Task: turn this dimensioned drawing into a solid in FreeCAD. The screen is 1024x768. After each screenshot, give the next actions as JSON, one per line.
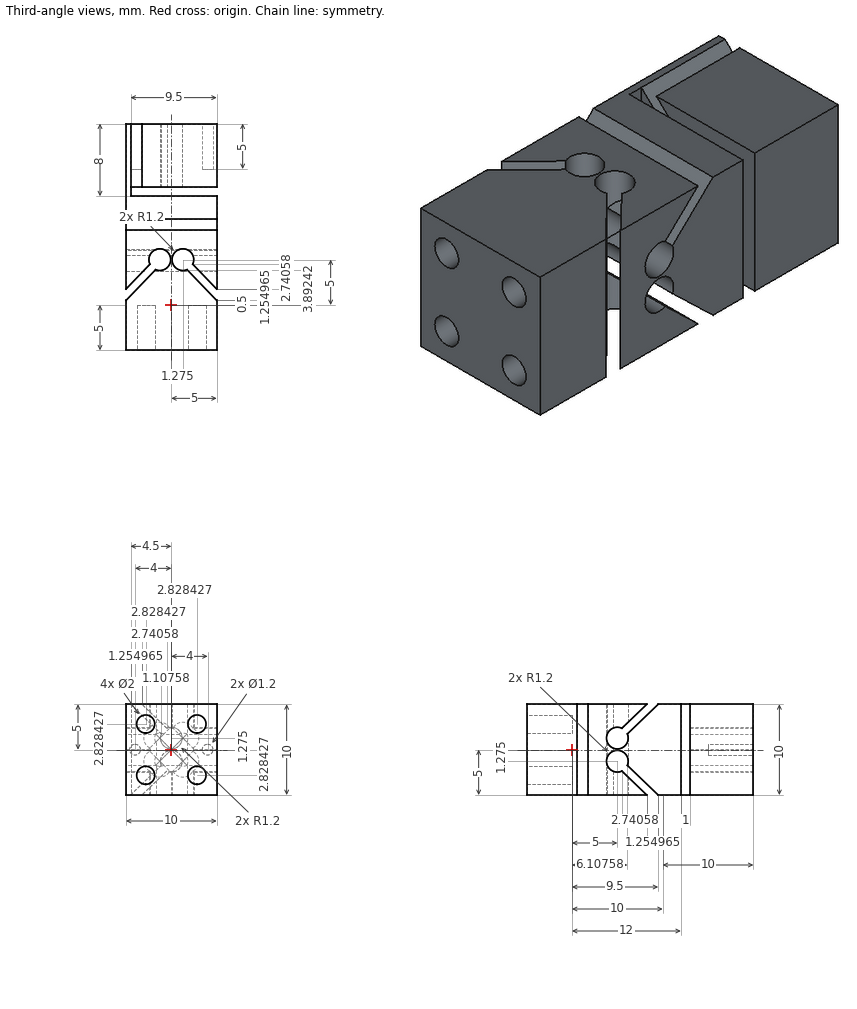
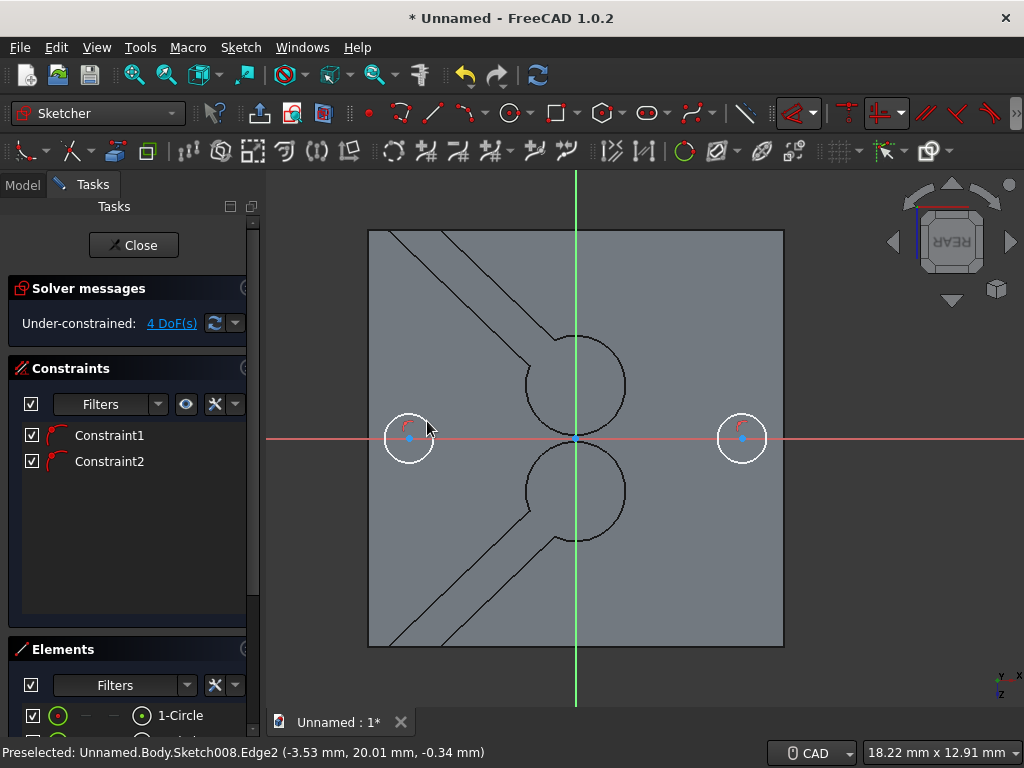
{"action": "left_click", "coordinate": [759, 421]}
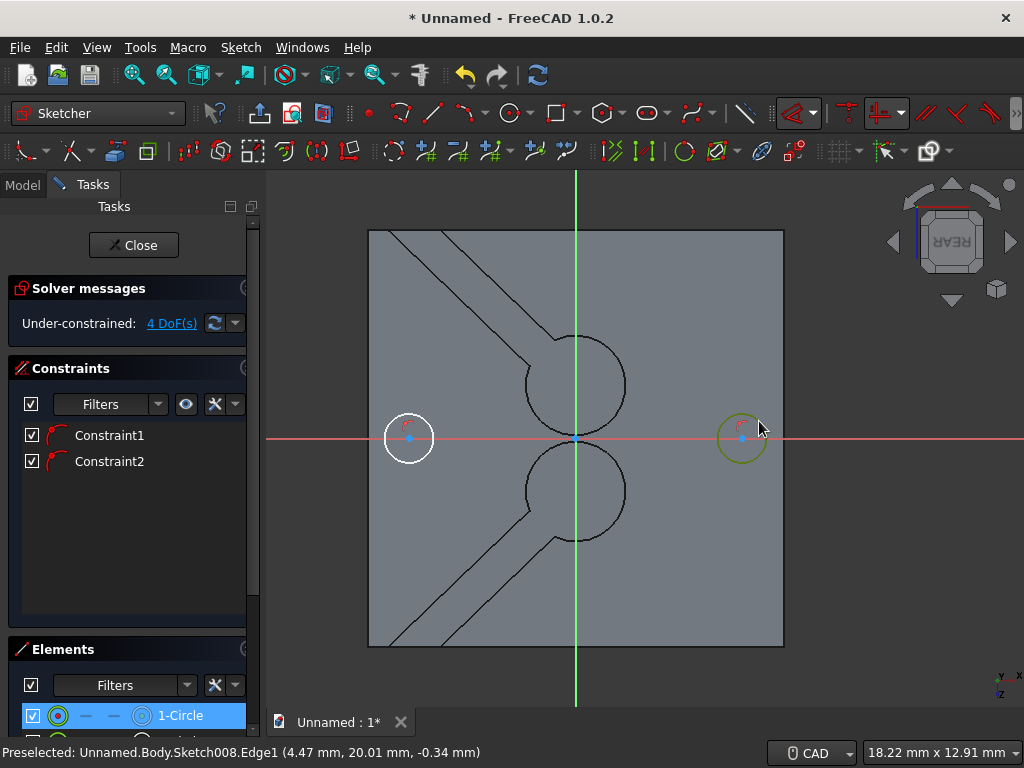
{"action": "left_click", "coordinate": [426, 421]}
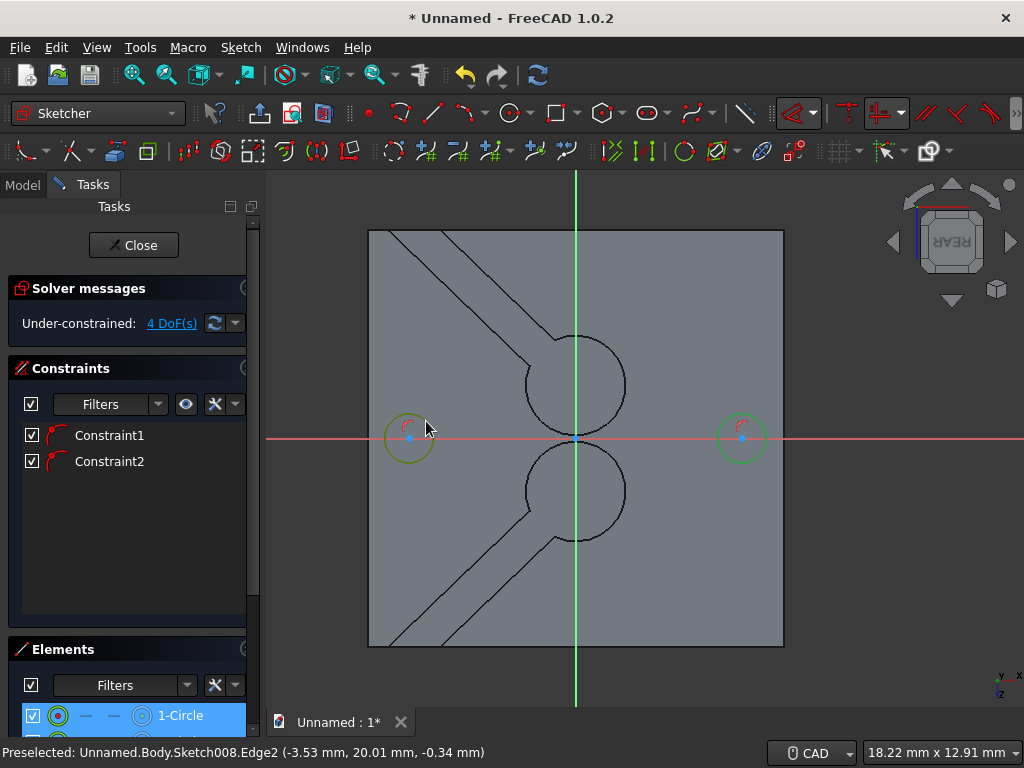
{"action": "key", "text": "e"}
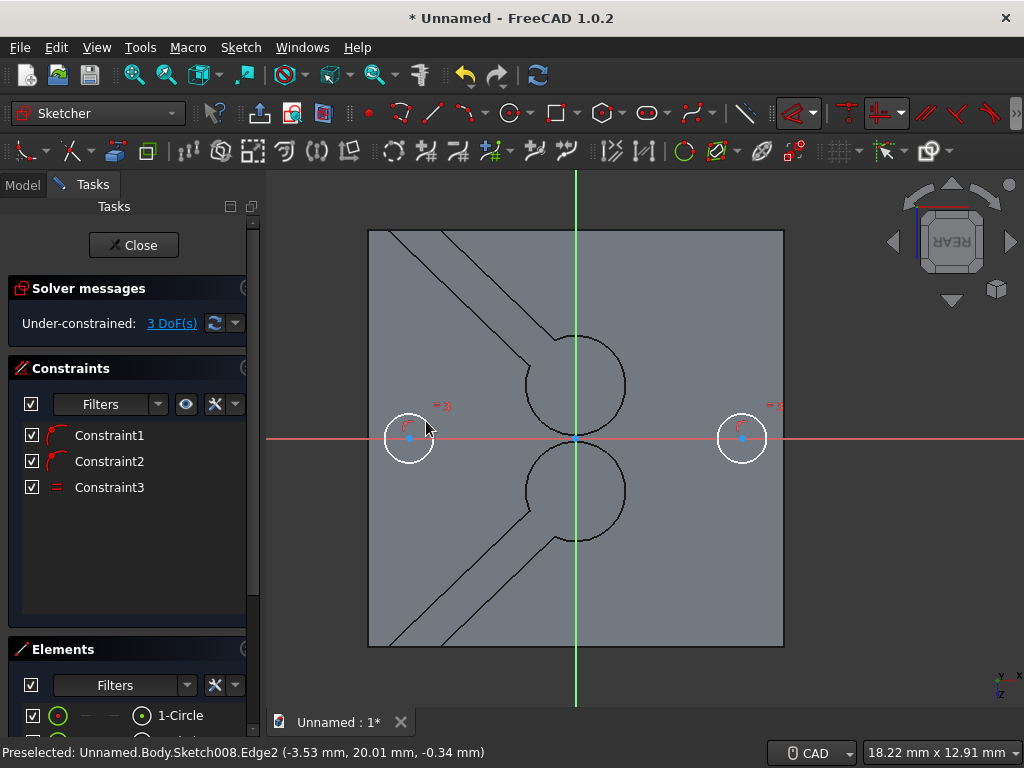
{"action": "left_click", "coordinate": [759, 421]}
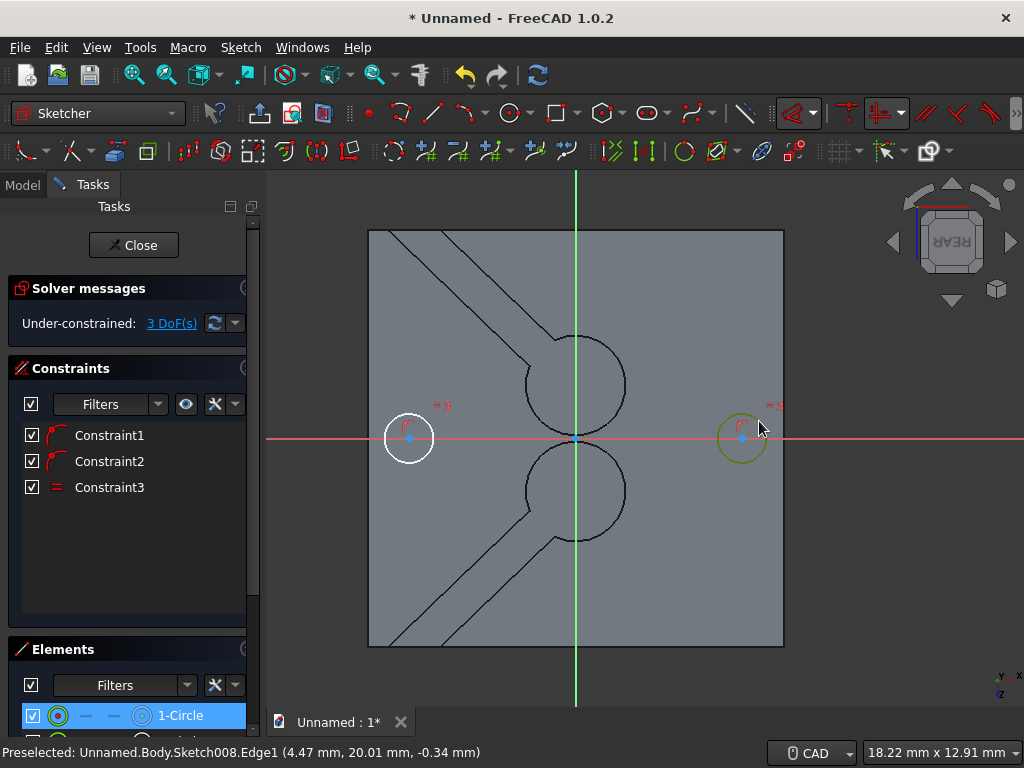
{"action": "left_click", "coordinate": [816, 114]}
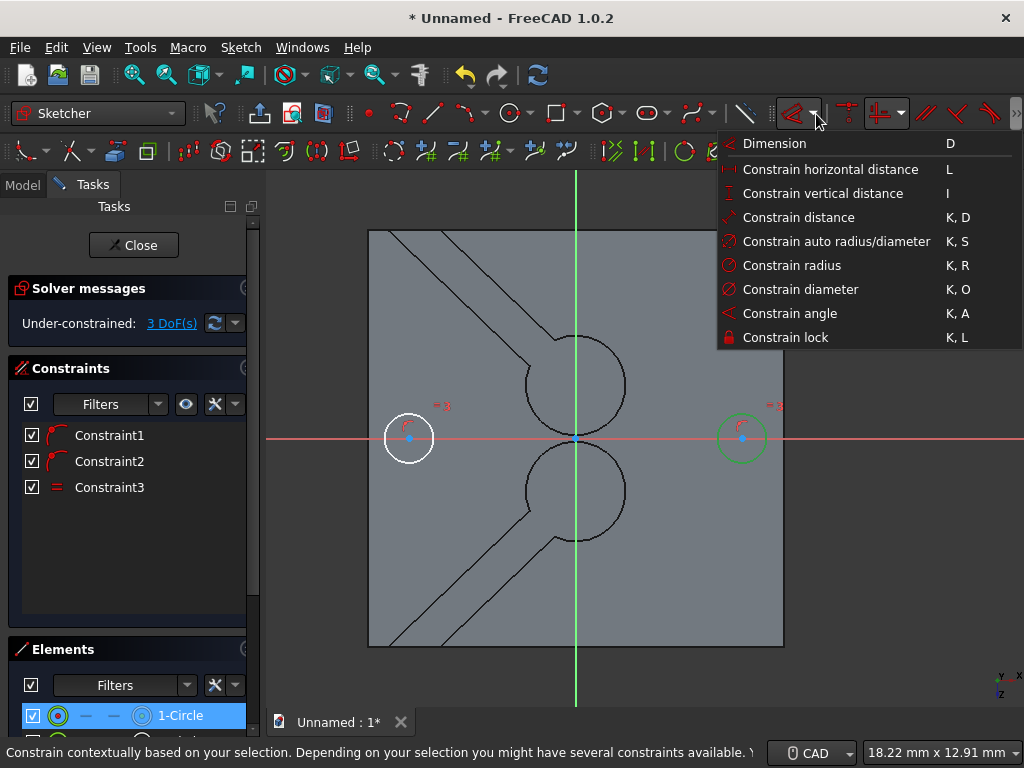
{"action": "left_click", "coordinate": [870, 289]}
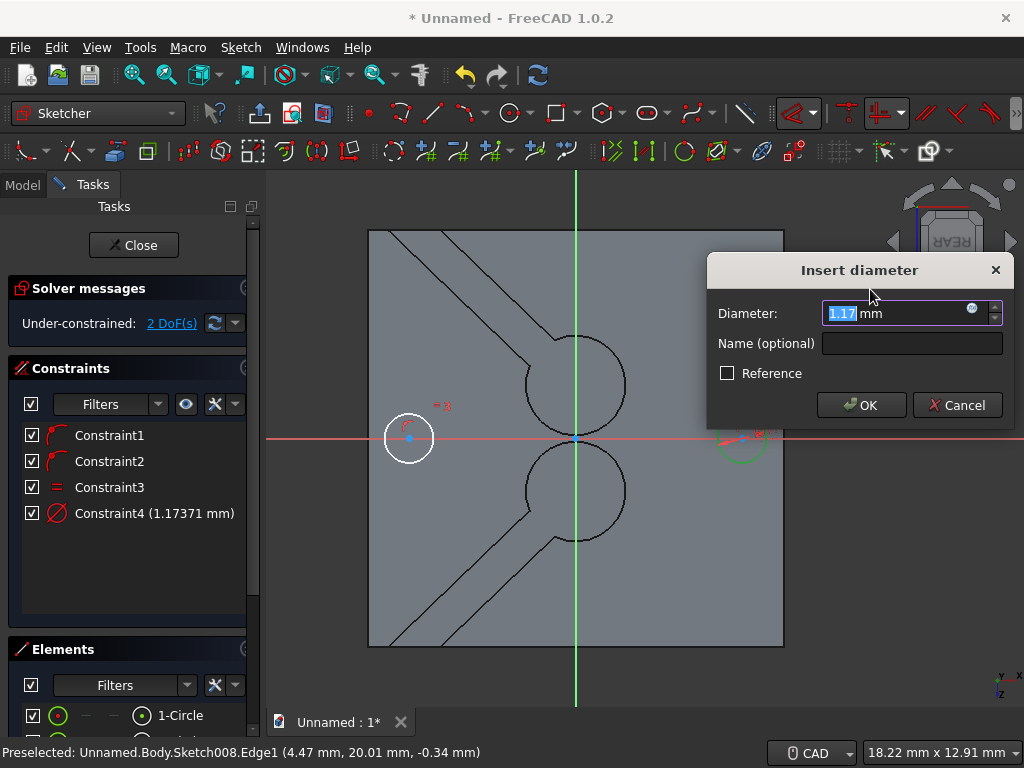
{"action": "type", "text": "1.2"}
{"action": "key", "text": "Return"}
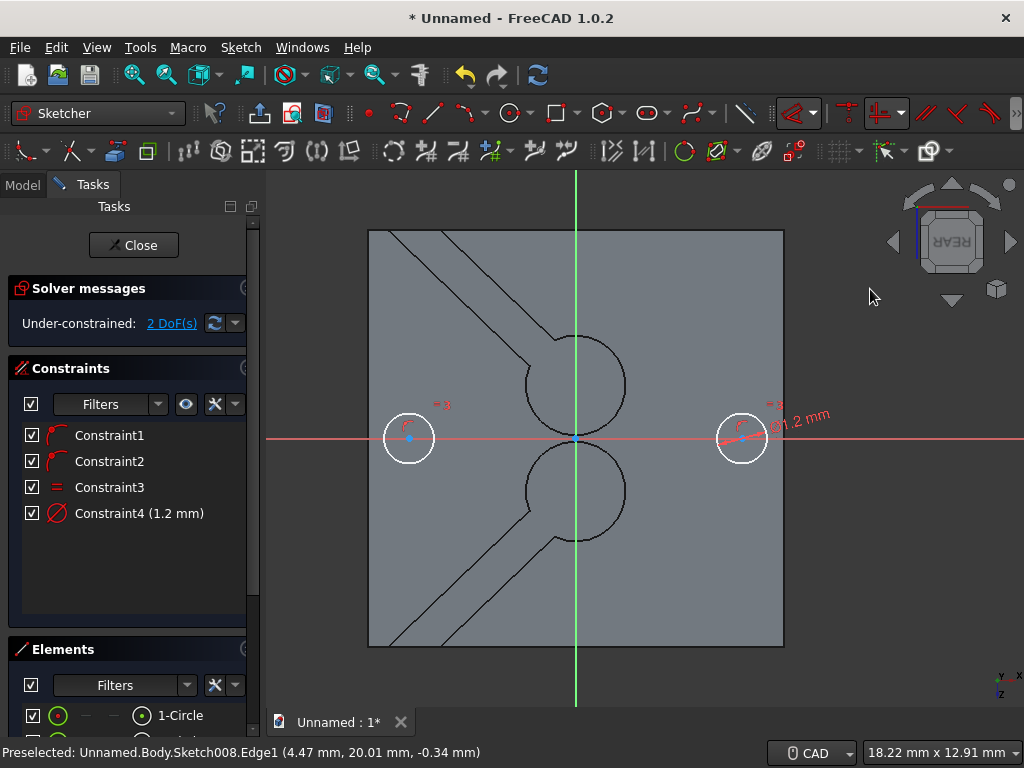
{"action": "left_click", "coordinate": [742, 438]}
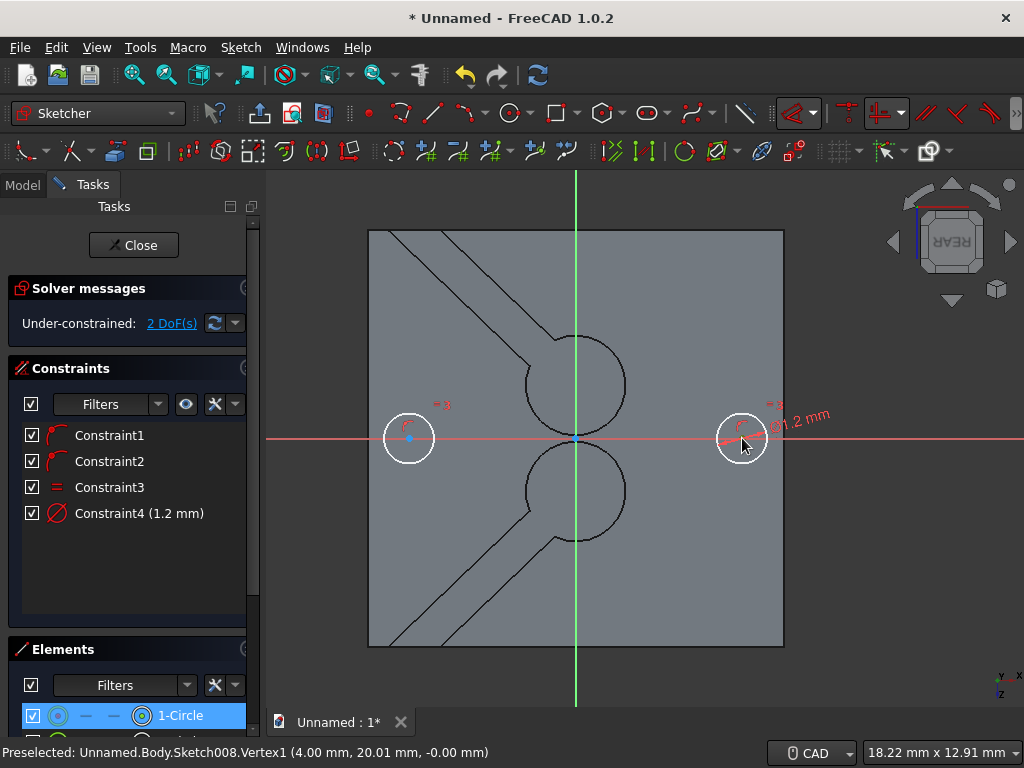
{"action": "key", "text": "l"}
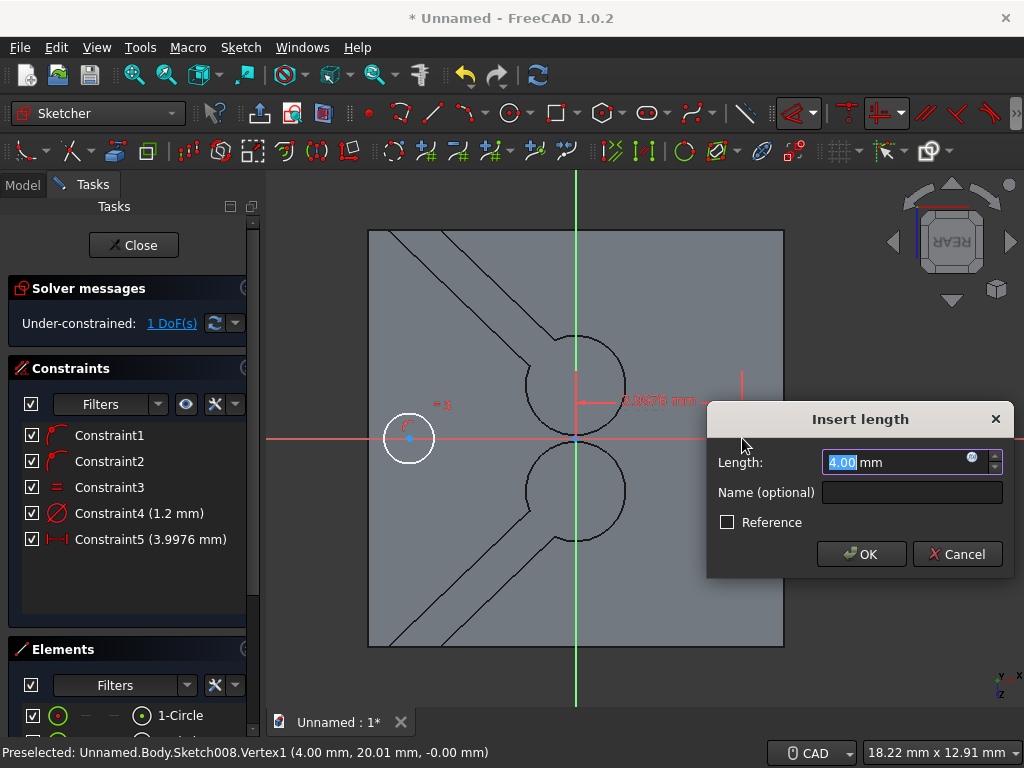
{"action": "type", "text": "4"}
{"action": "key", "text": "Return"}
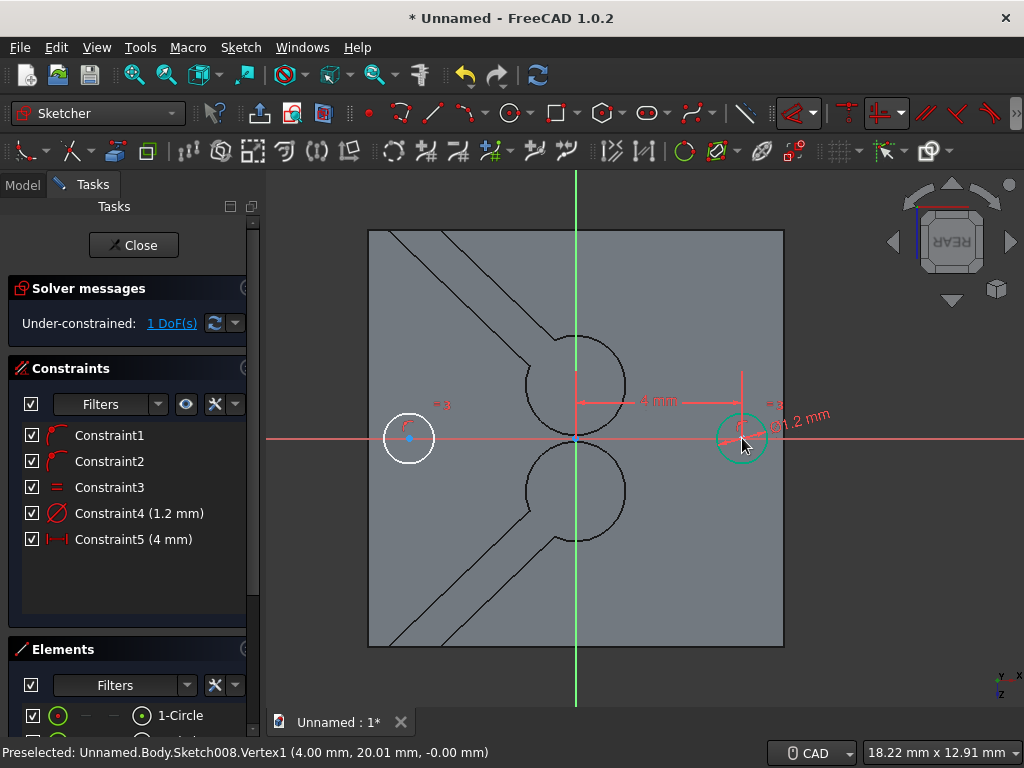
{"action": "left_click", "coordinate": [409, 438]}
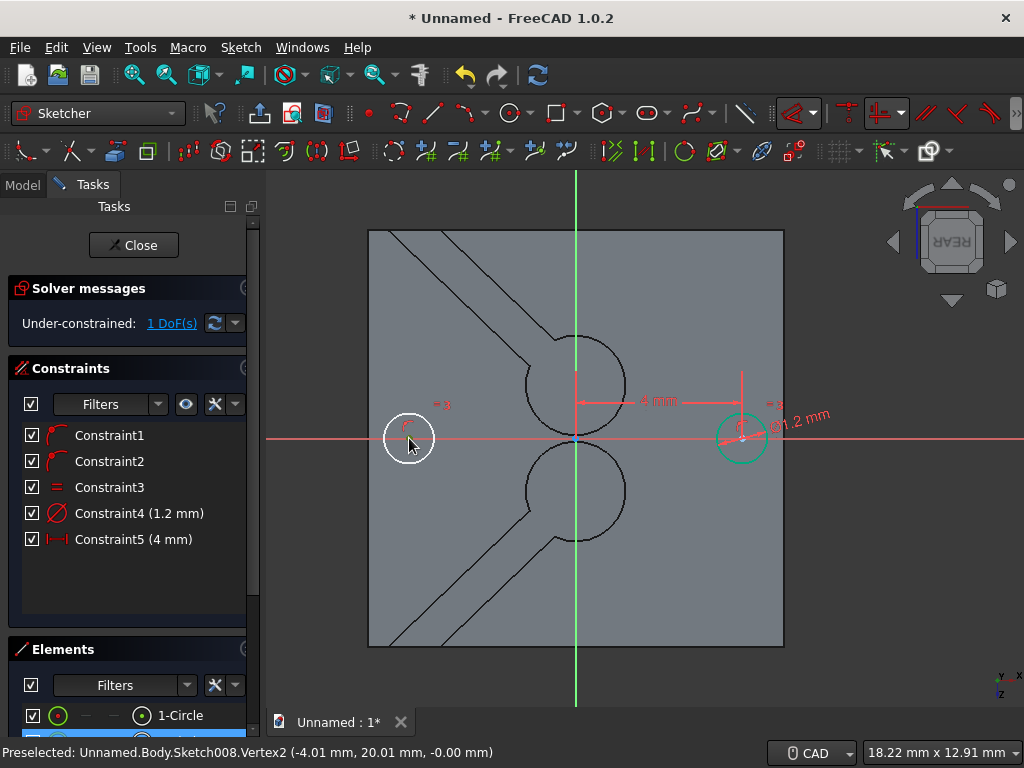
{"action": "key", "text": "l"}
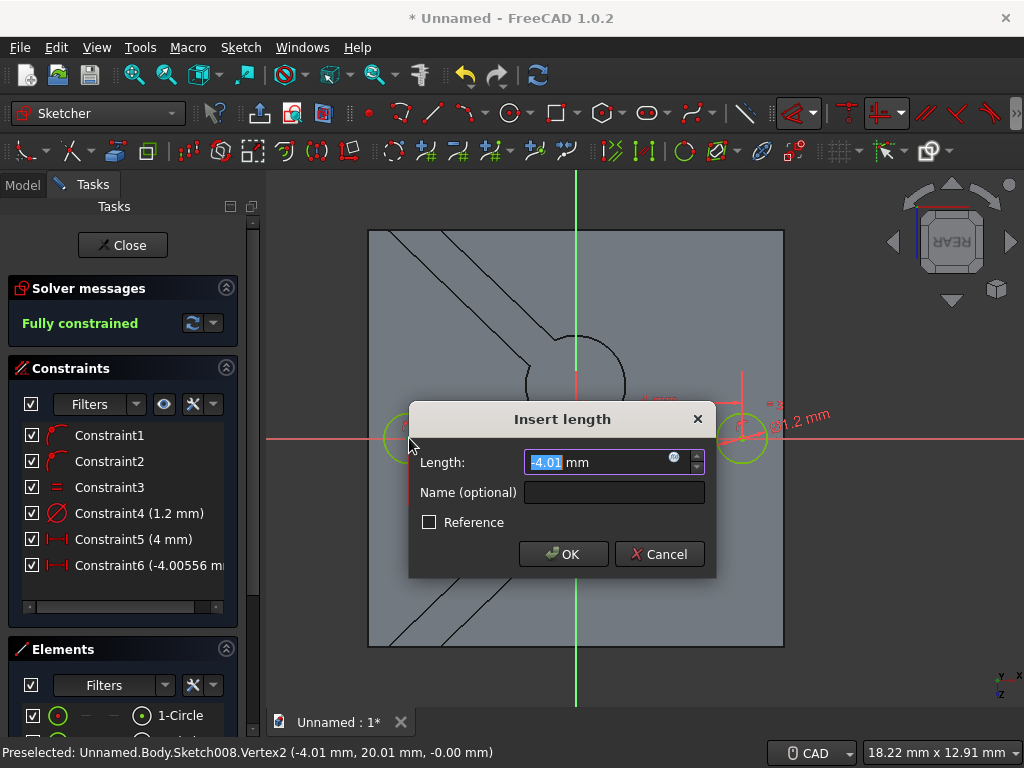
{"action": "type", "text": "-4"}
{"action": "key", "text": "Return"}